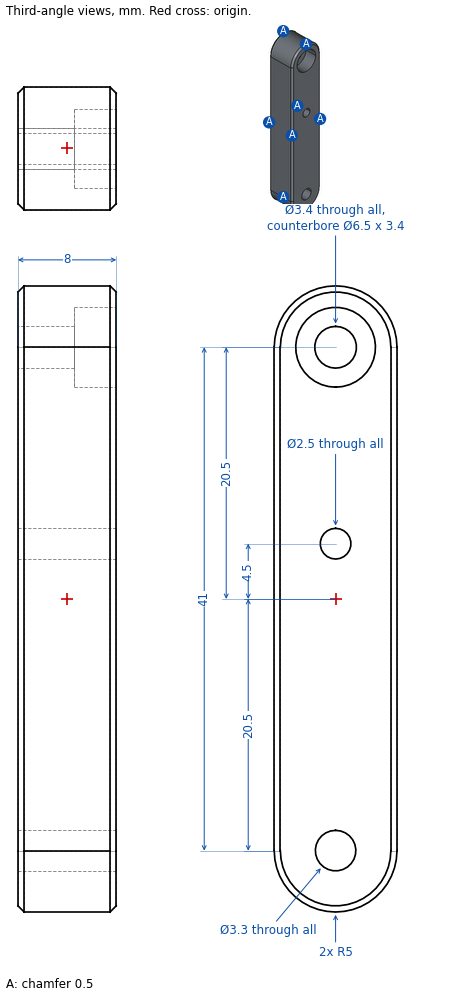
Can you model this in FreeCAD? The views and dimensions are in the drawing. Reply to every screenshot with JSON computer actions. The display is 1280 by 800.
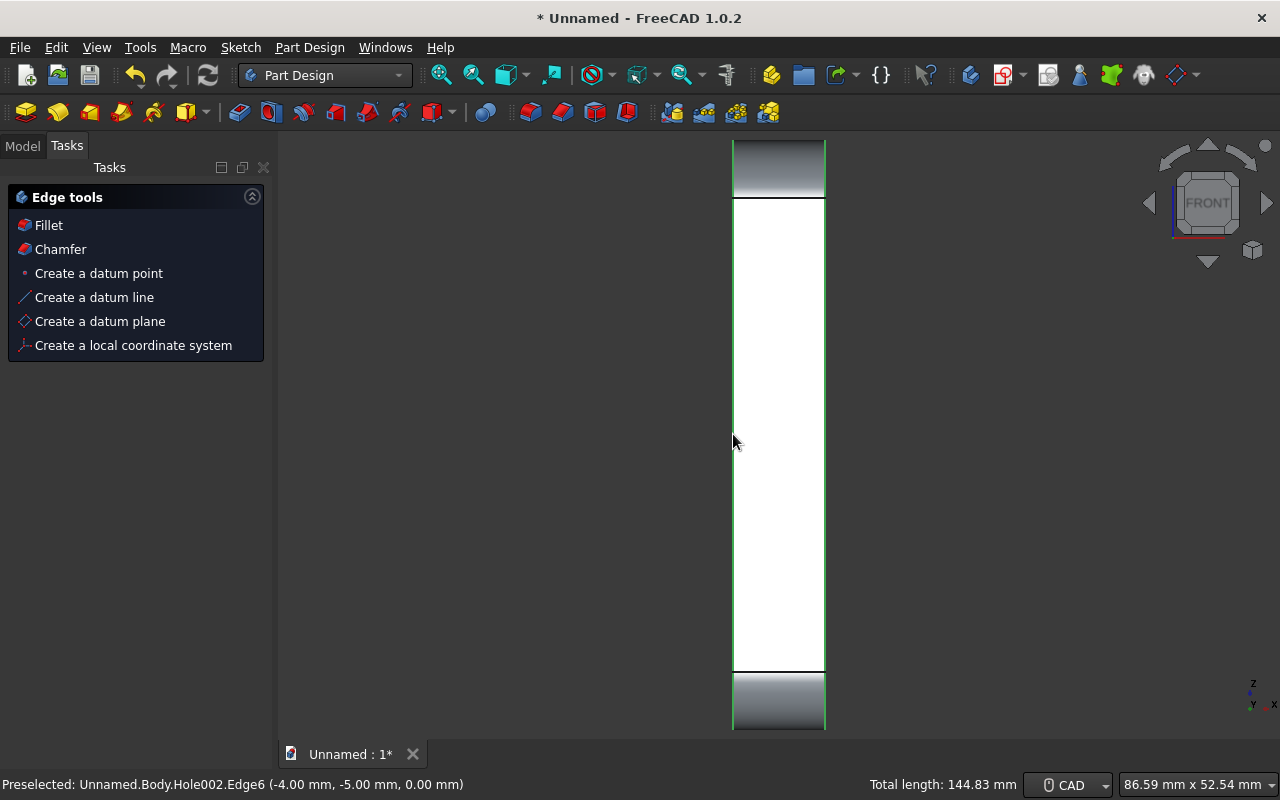
{"action": "key", "text": "3"}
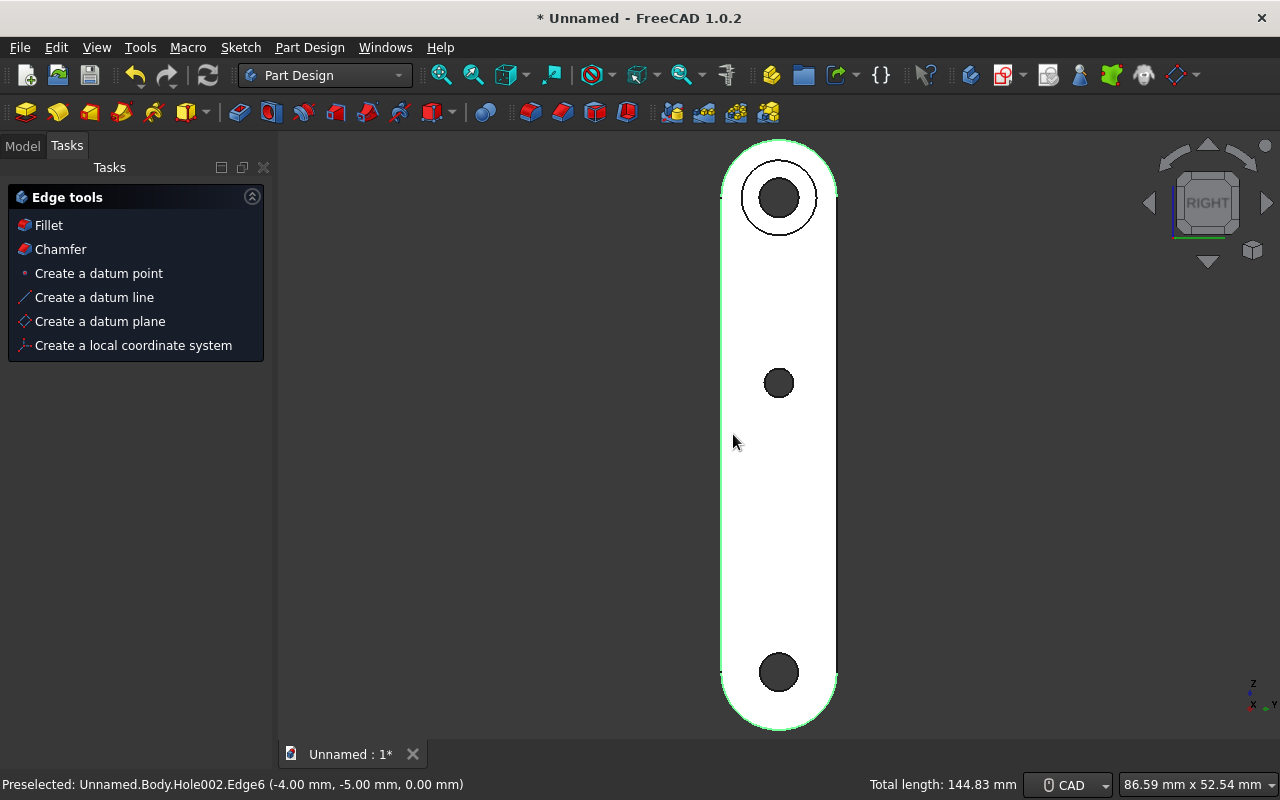
{"action": "left_click", "coordinate": [837, 434], "text": "ctrl"}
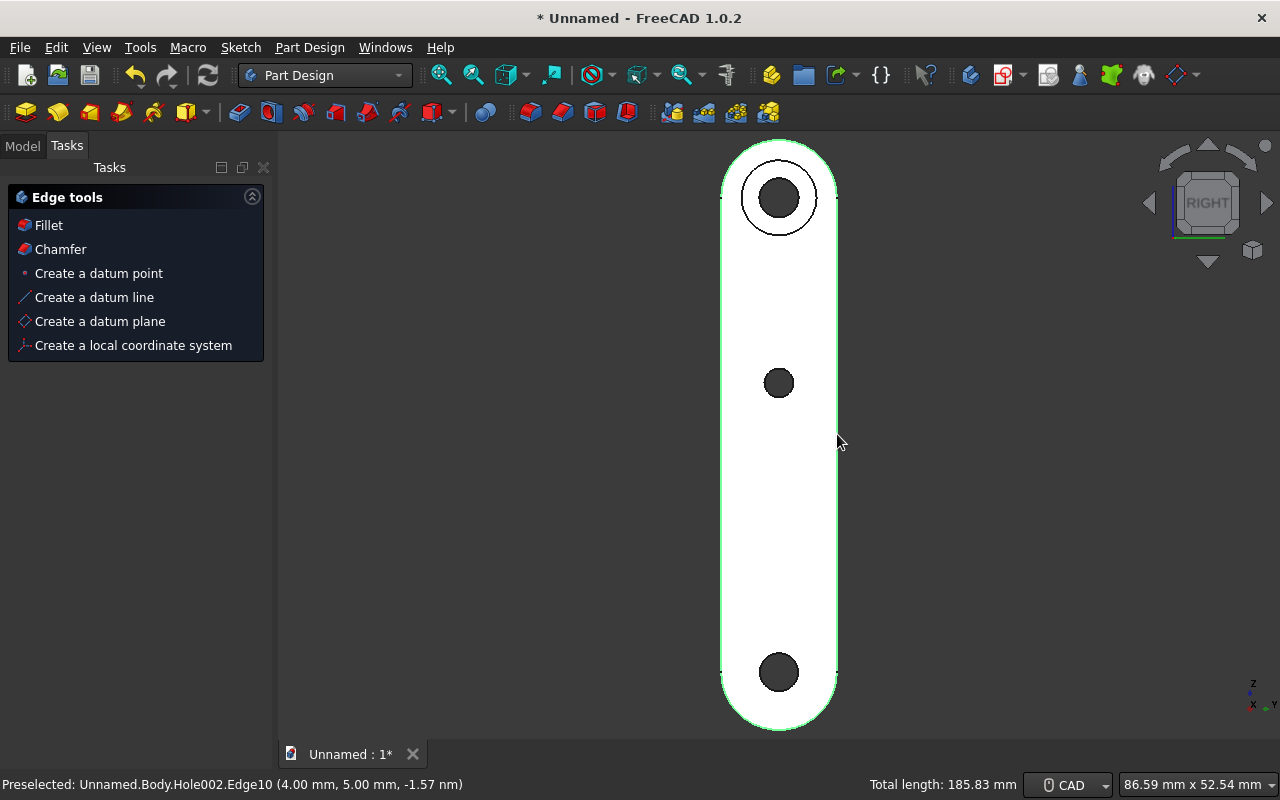
{"action": "key", "text": "5"}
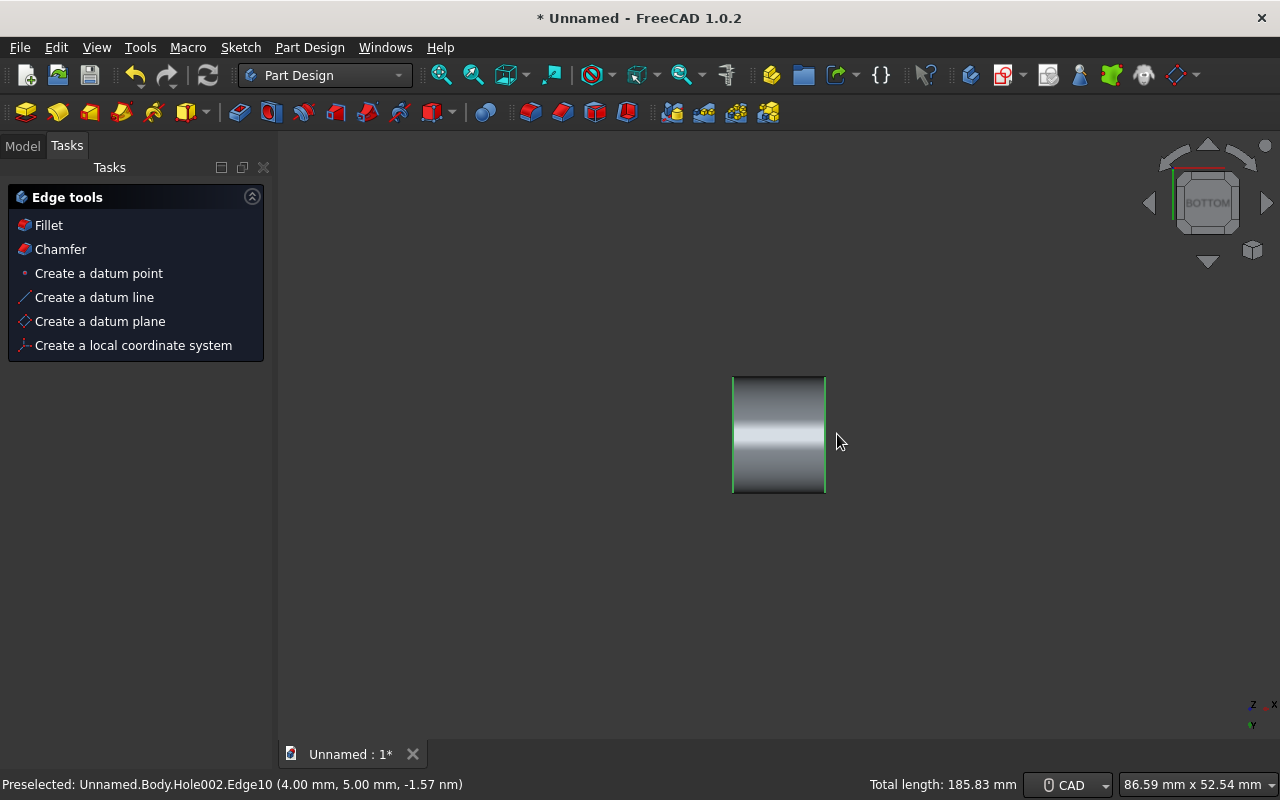
{"action": "key", "text": "v f"}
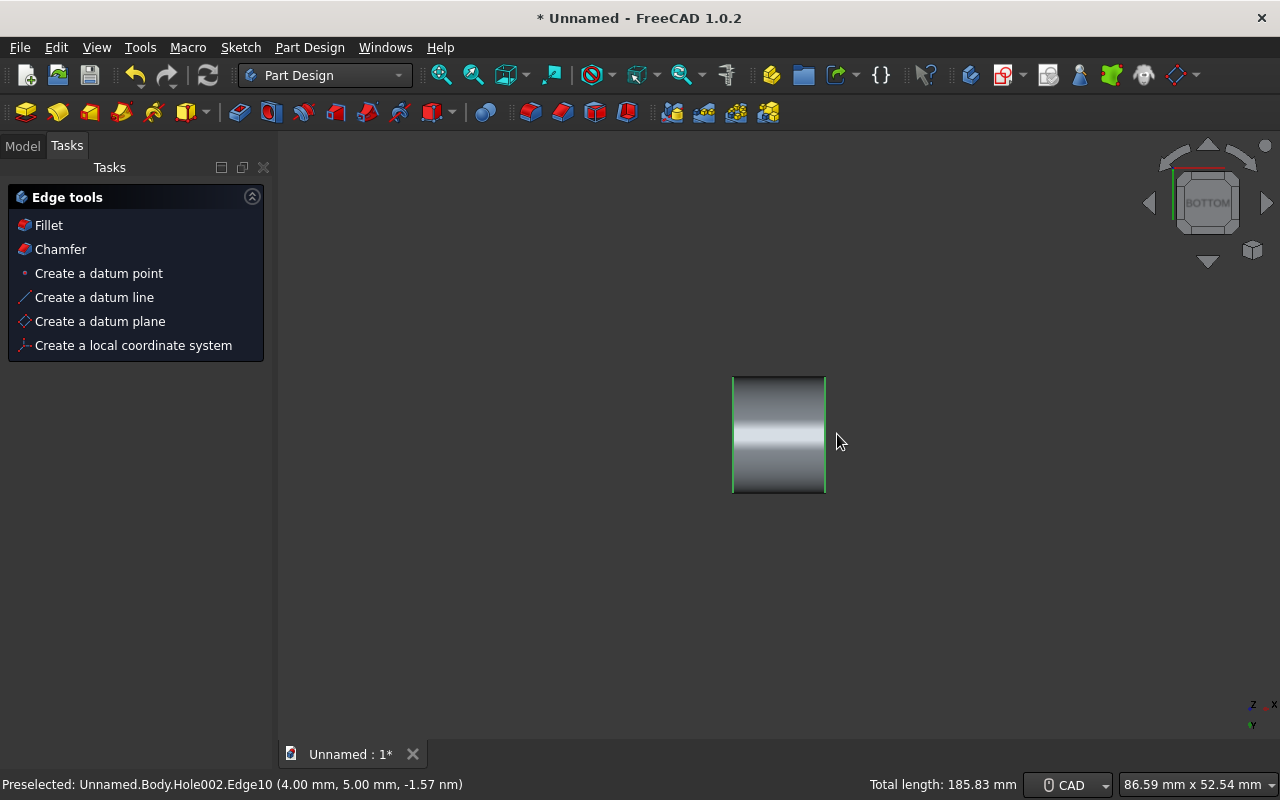
{"action": "key", "text": "4"}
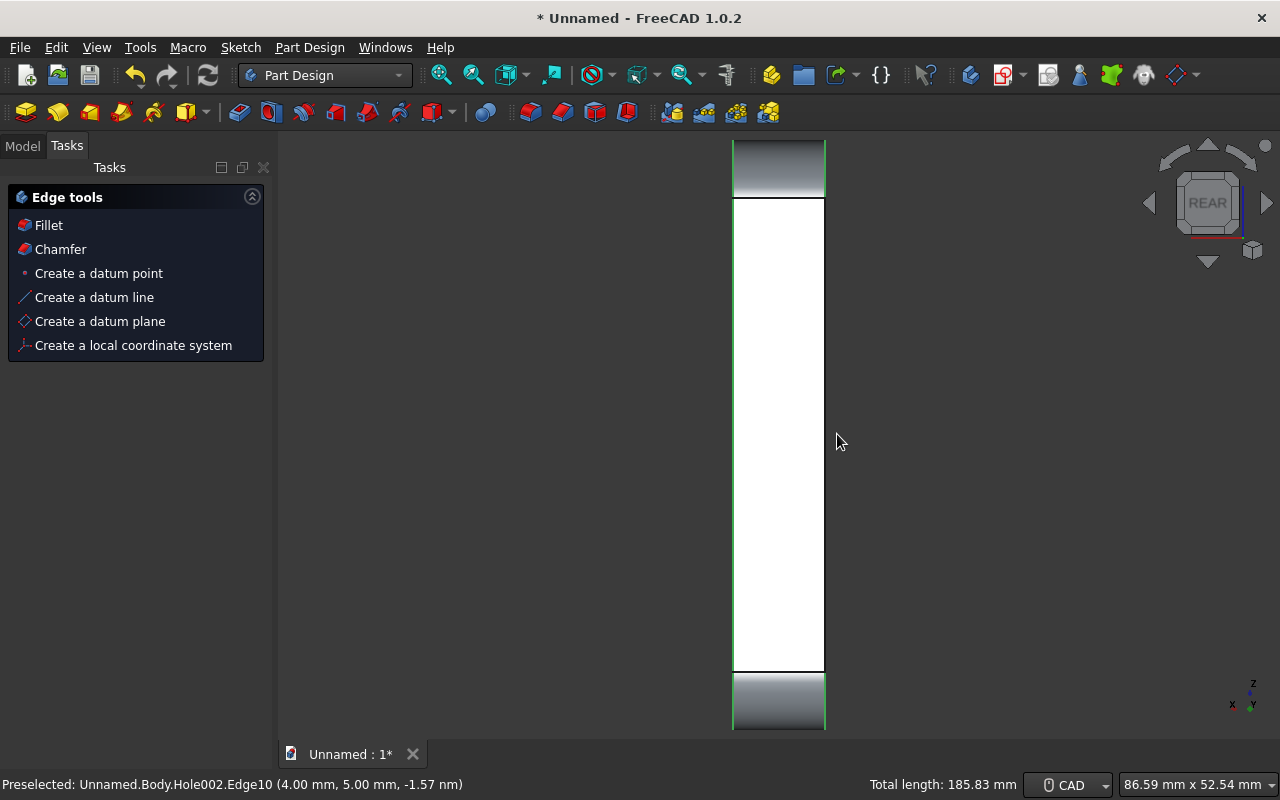
{"action": "left_click", "coordinate": [825, 434], "text": "ctrl"}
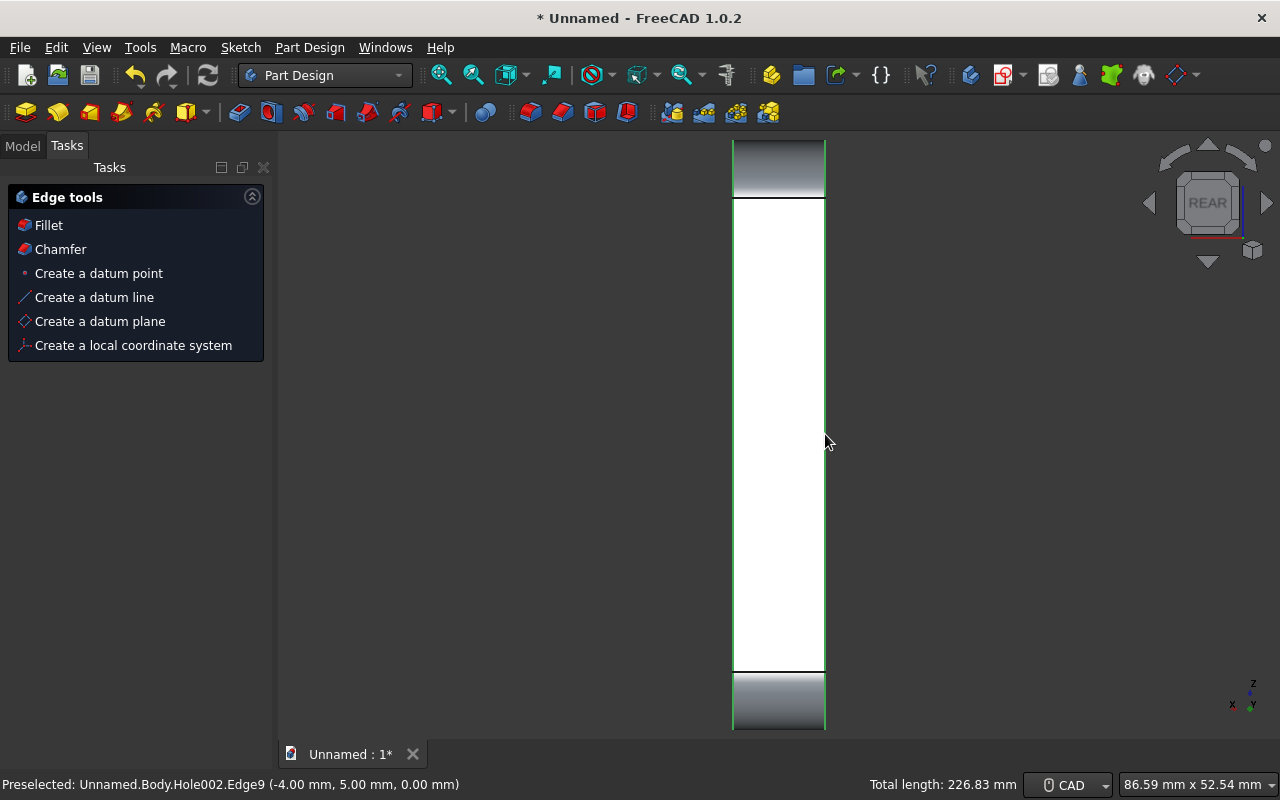
{"action": "left_click", "coordinate": [564, 112]}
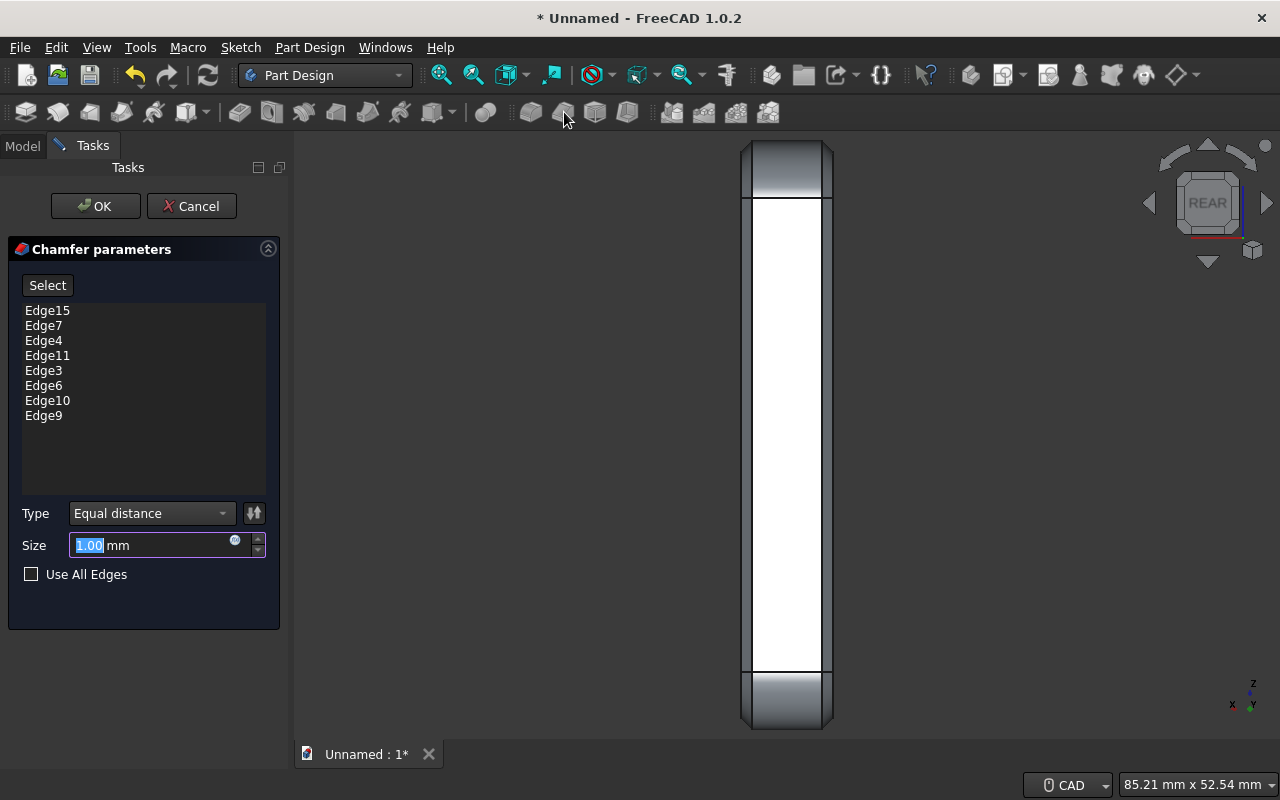
{"action": "type", "text": "0.5"}
{"action": "key", "text": "Tab"}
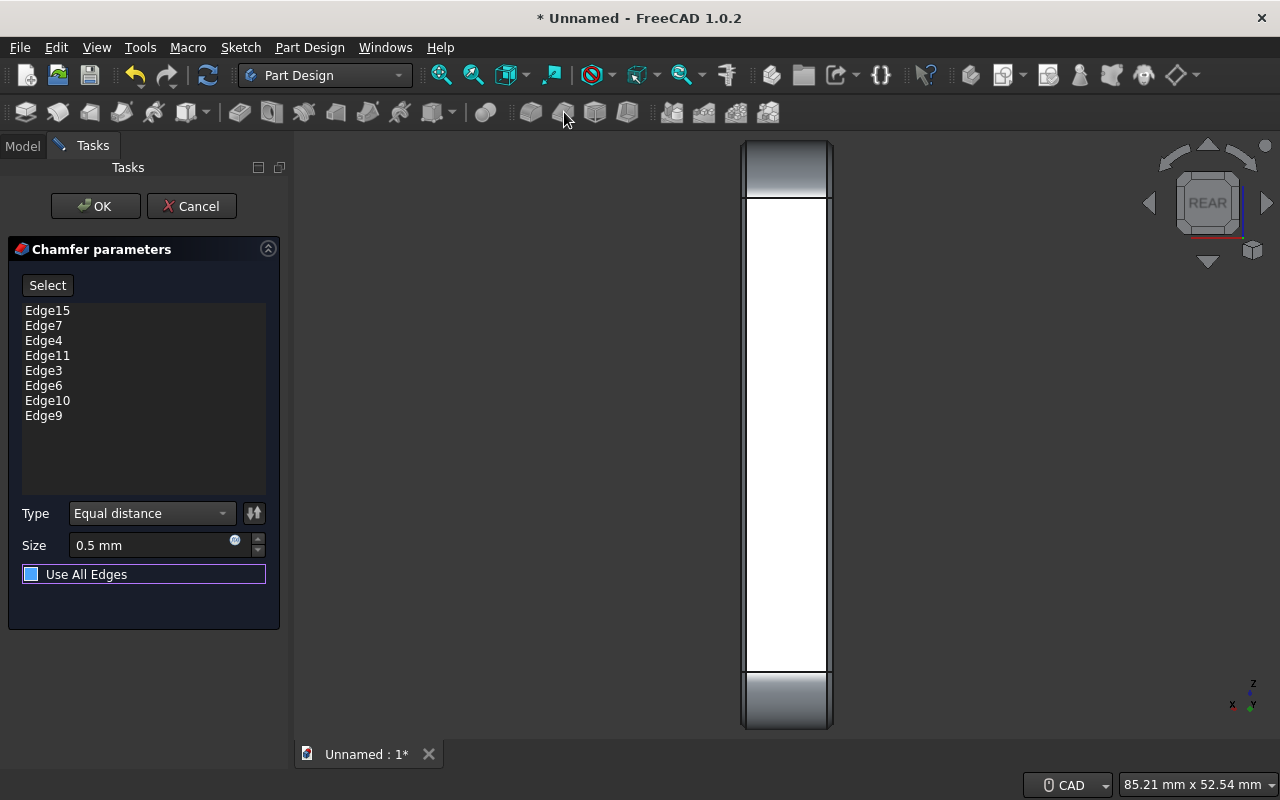
{"action": "left_click", "coordinate": [96, 206]}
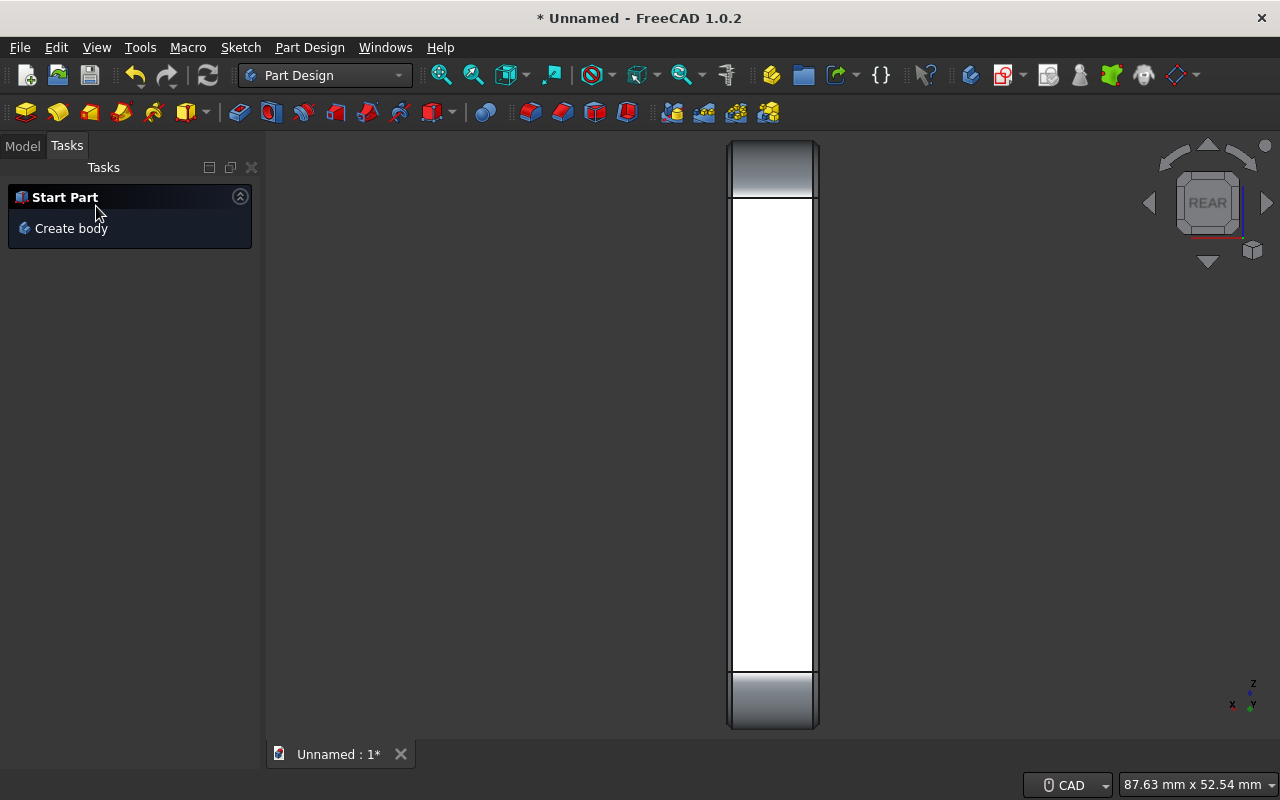
{"action": "key", "text": "0"}